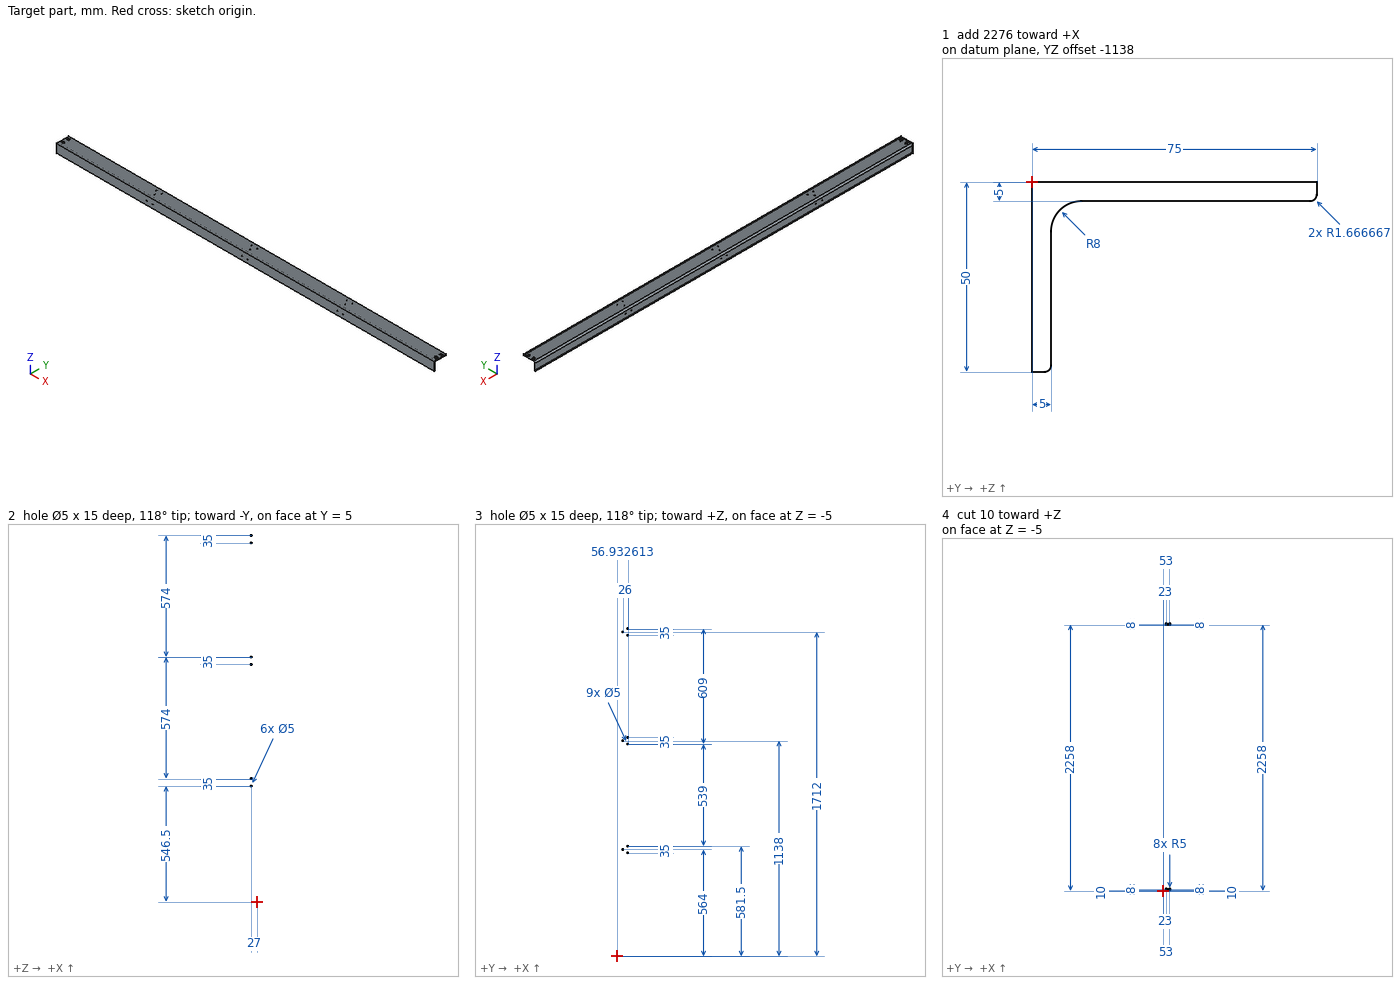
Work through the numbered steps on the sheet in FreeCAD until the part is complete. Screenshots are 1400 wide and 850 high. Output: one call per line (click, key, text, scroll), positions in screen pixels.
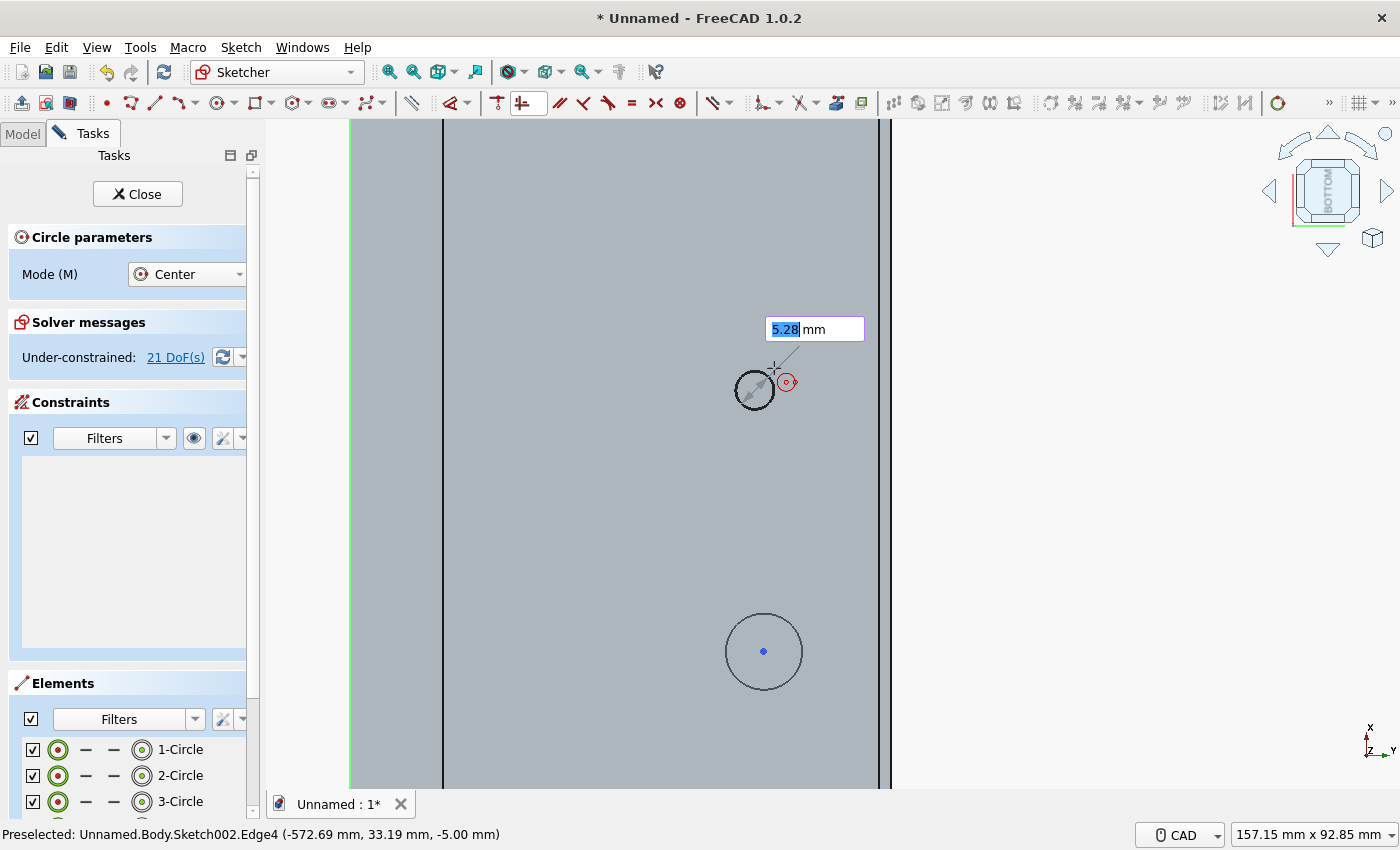
click(773, 361)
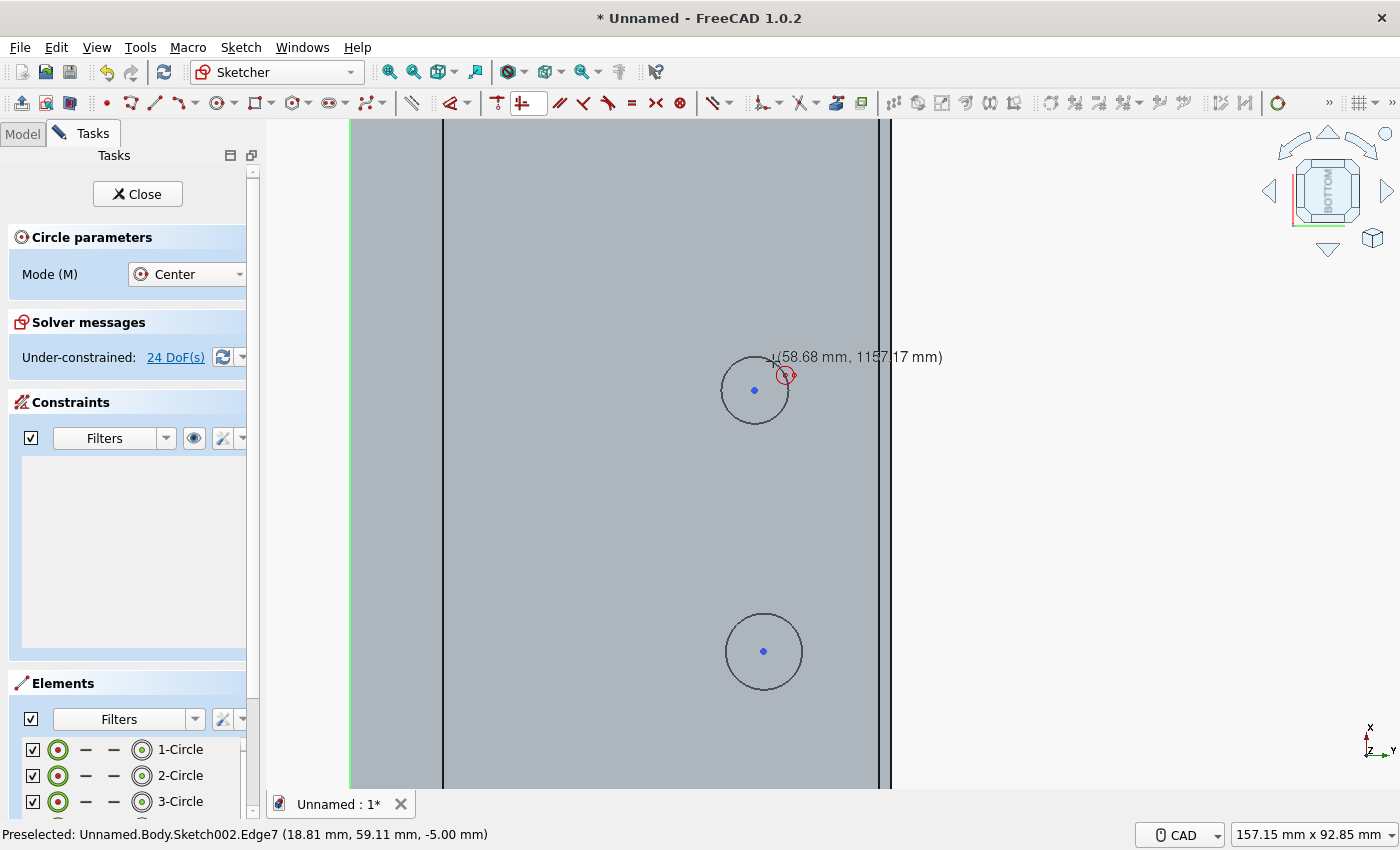
scroll(573, 500, up, 2)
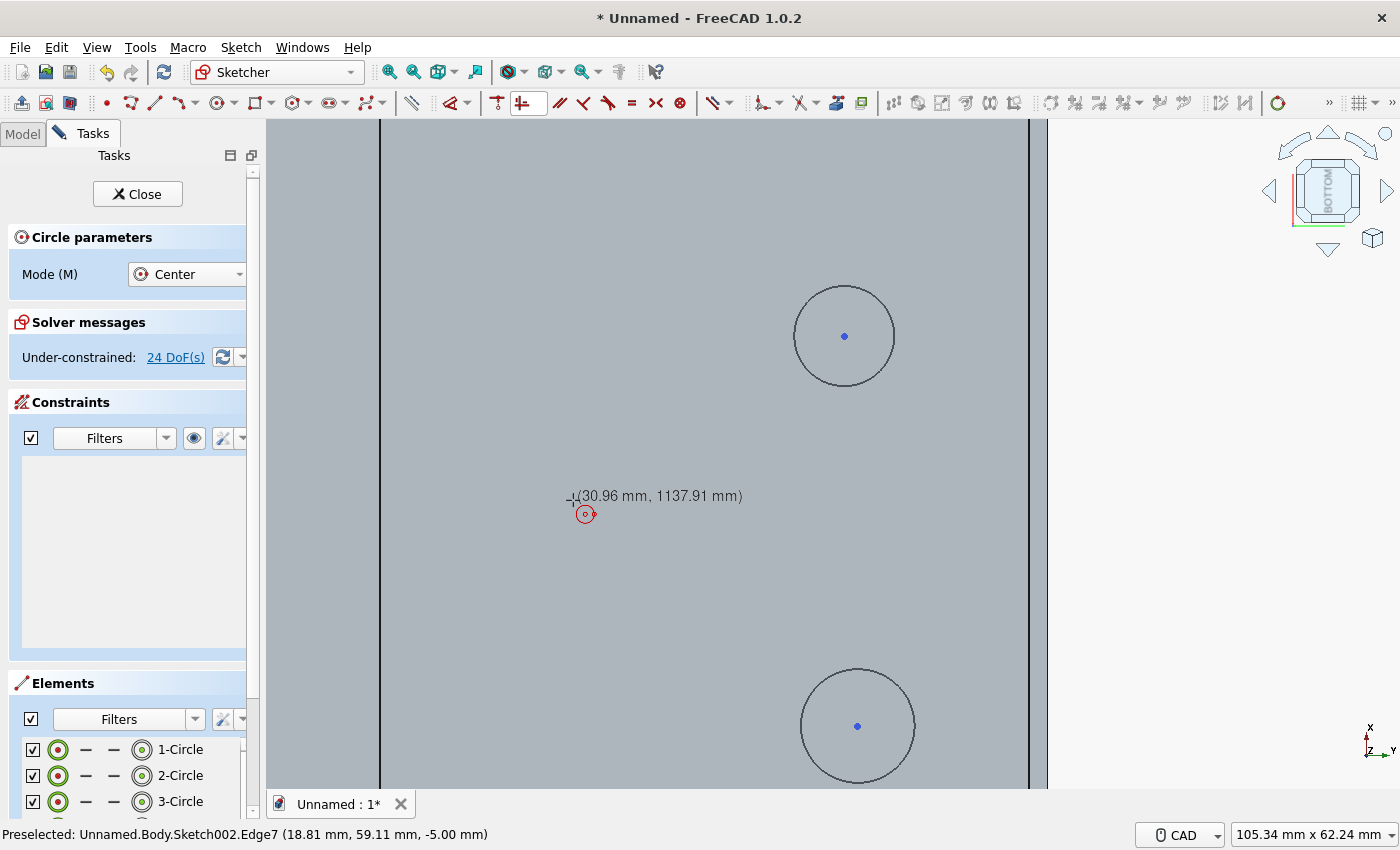
scroll(770, 370, down, 18)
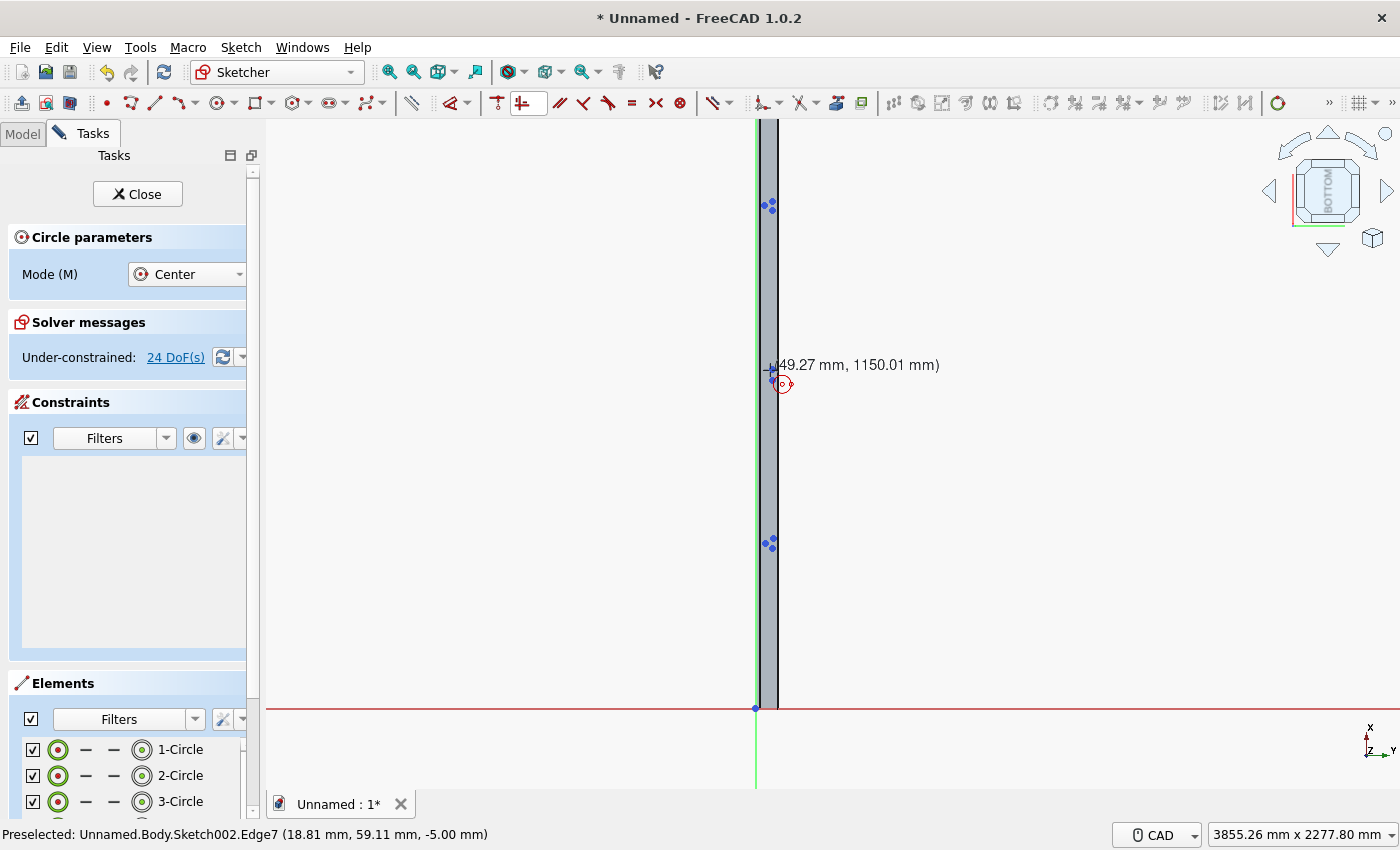
scroll(765, 374, up, 4)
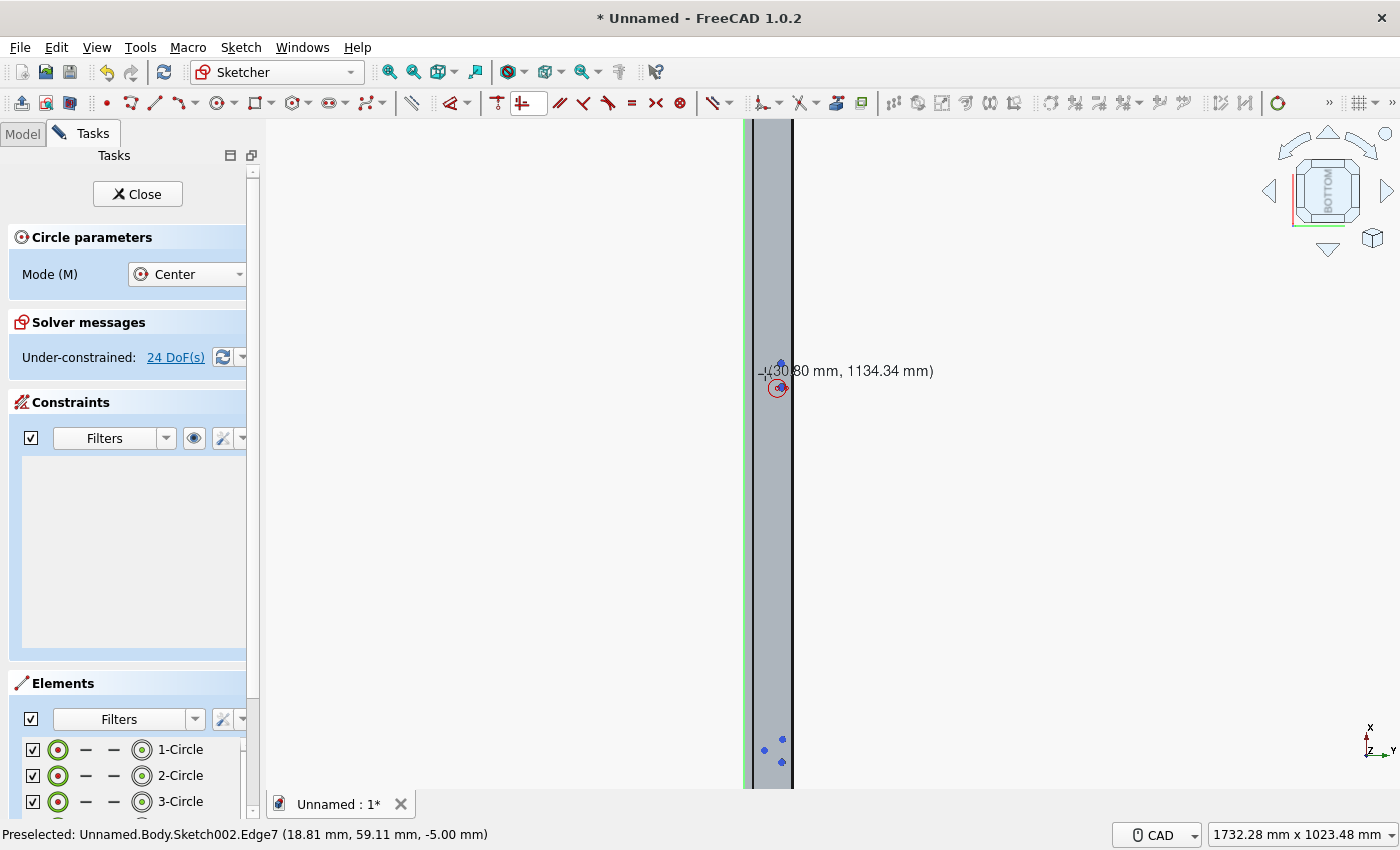
click(765, 373)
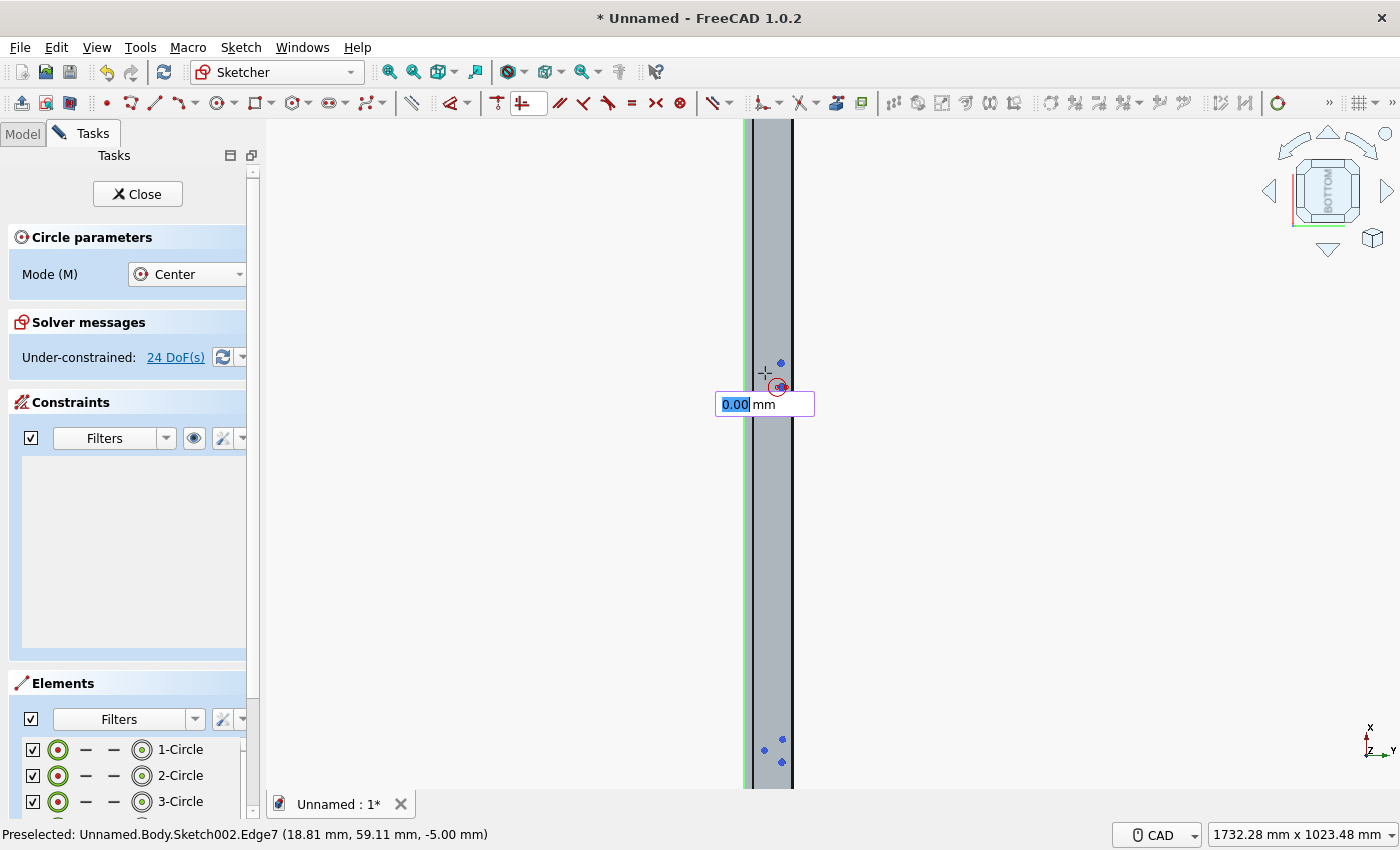
scroll(766, 372, up, 12)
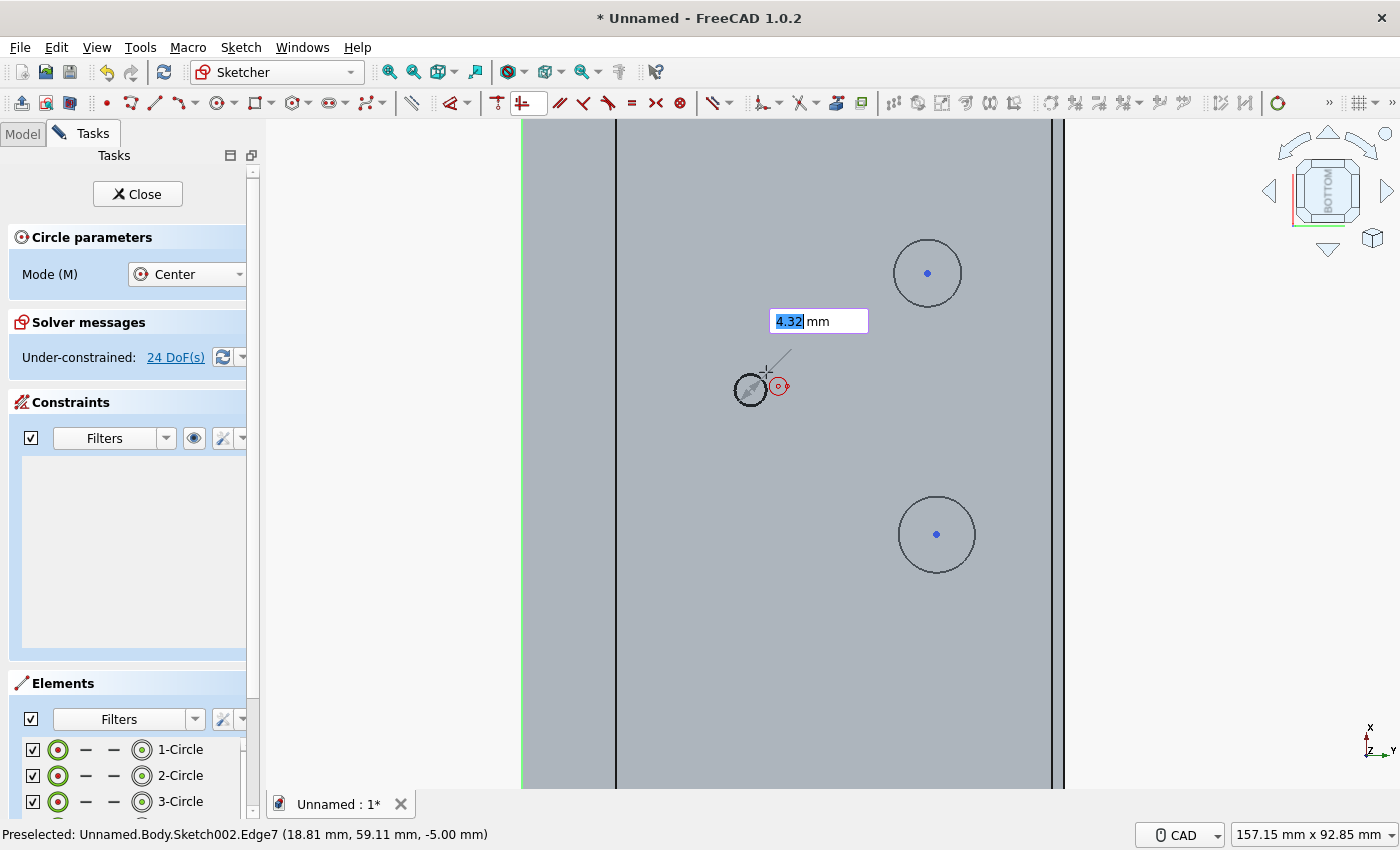
click(758, 370)
key(Escape)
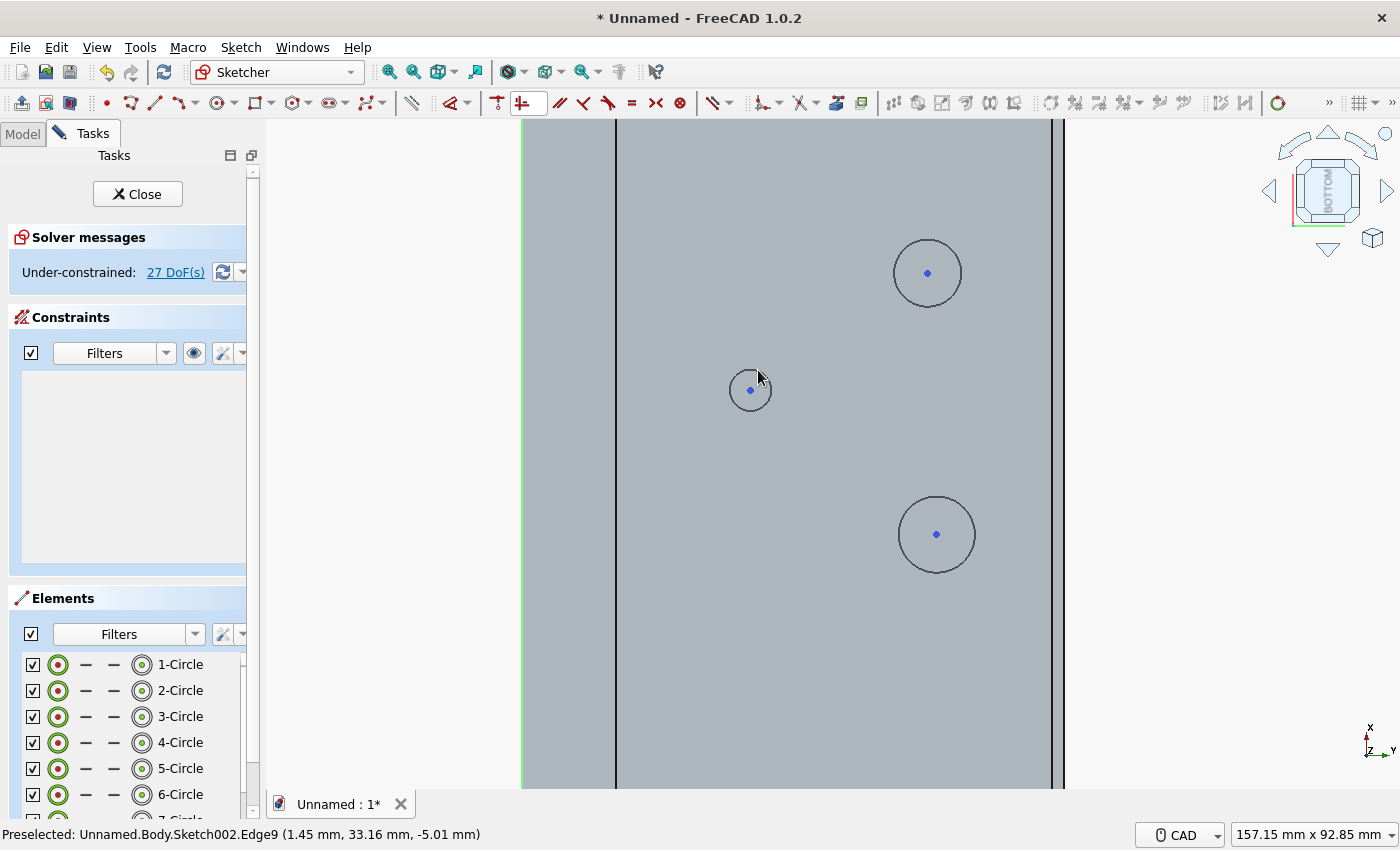
click(964, 508)